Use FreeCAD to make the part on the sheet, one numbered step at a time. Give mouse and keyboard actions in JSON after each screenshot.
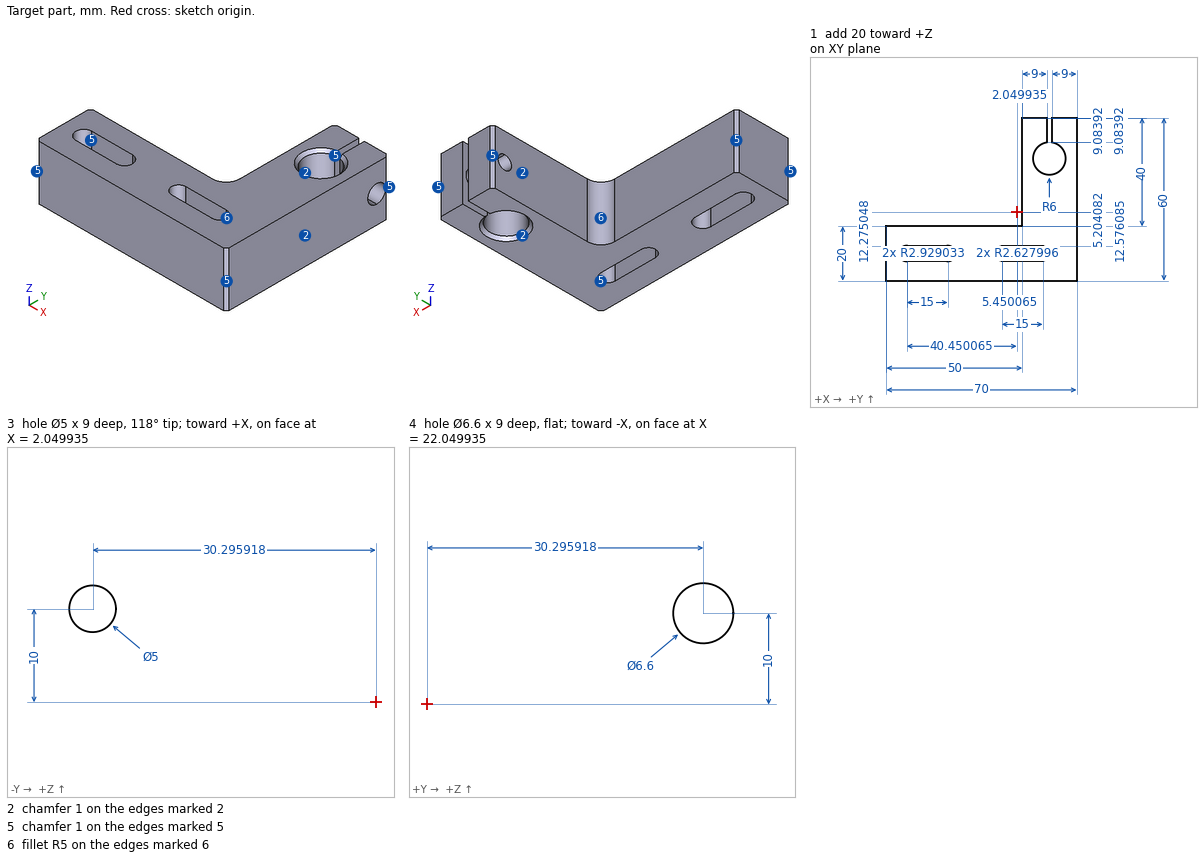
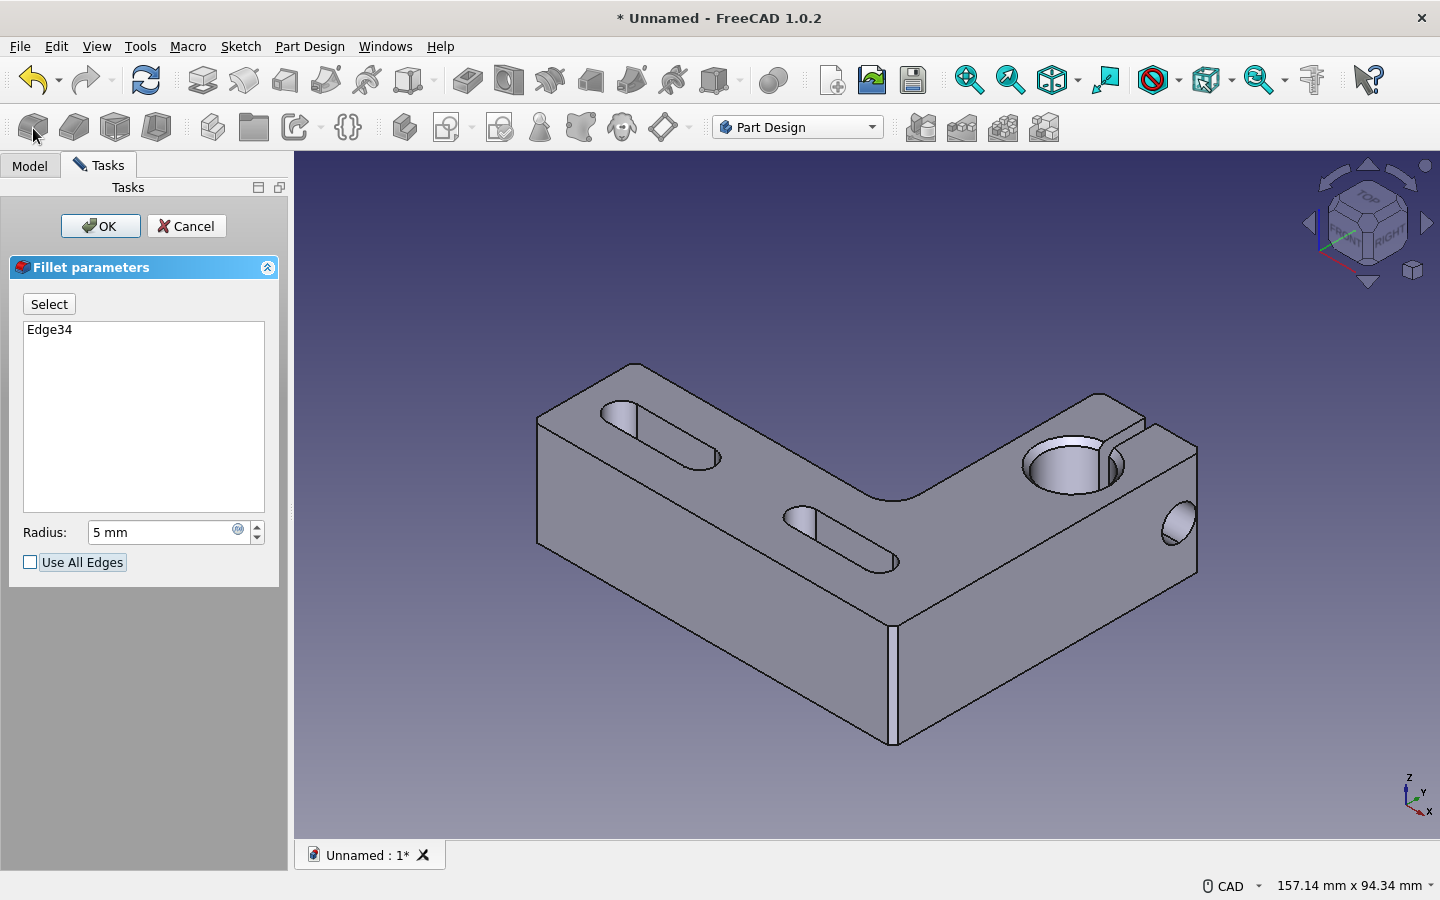
{"action": "left_click", "coordinate": [101, 226]}